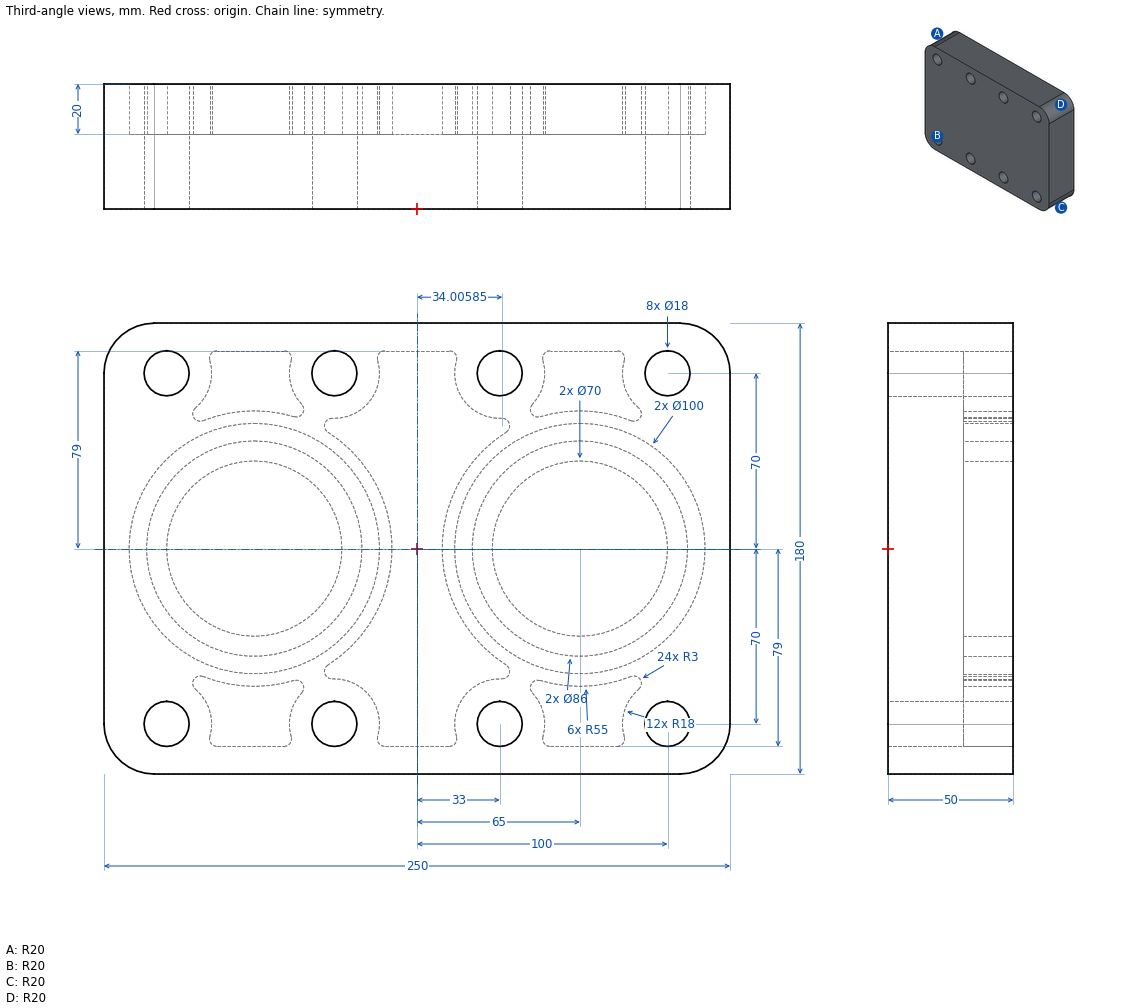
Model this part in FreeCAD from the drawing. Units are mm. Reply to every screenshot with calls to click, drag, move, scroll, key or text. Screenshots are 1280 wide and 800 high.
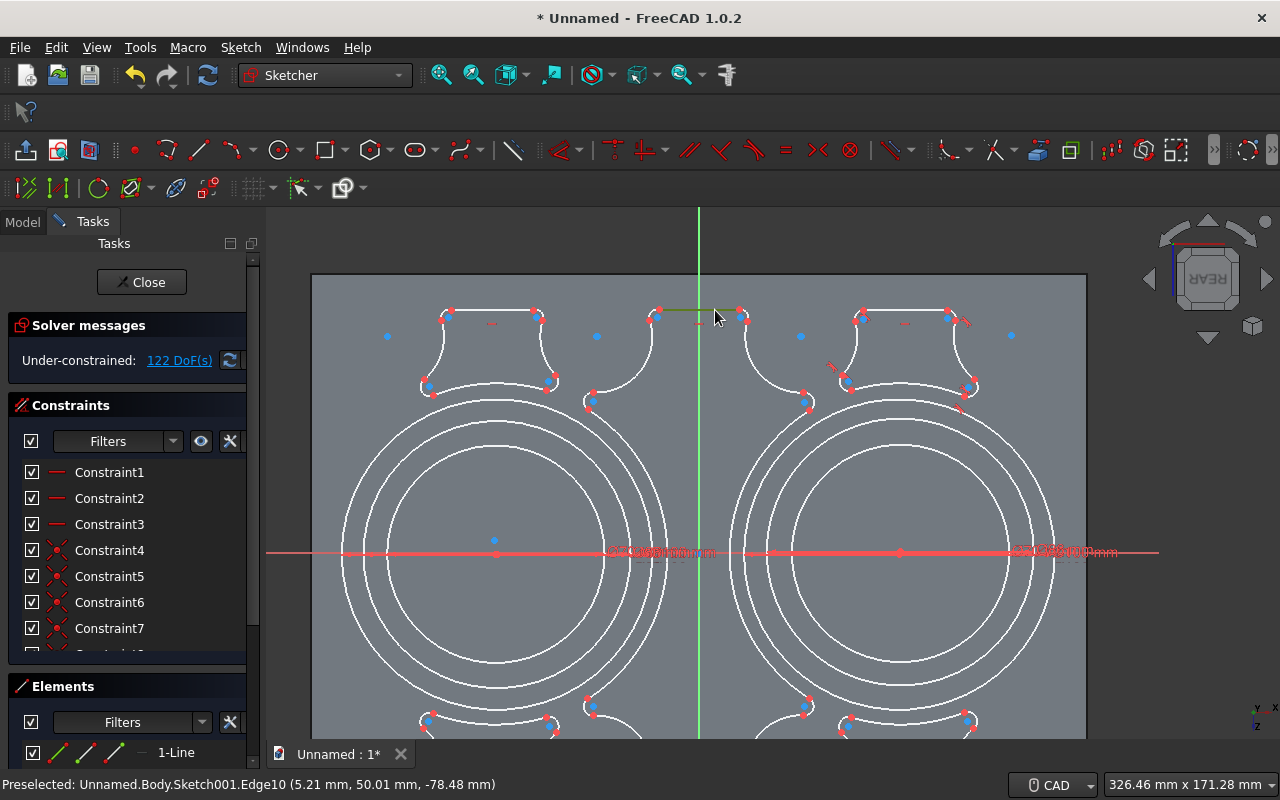
scroll(747, 313, up, 3)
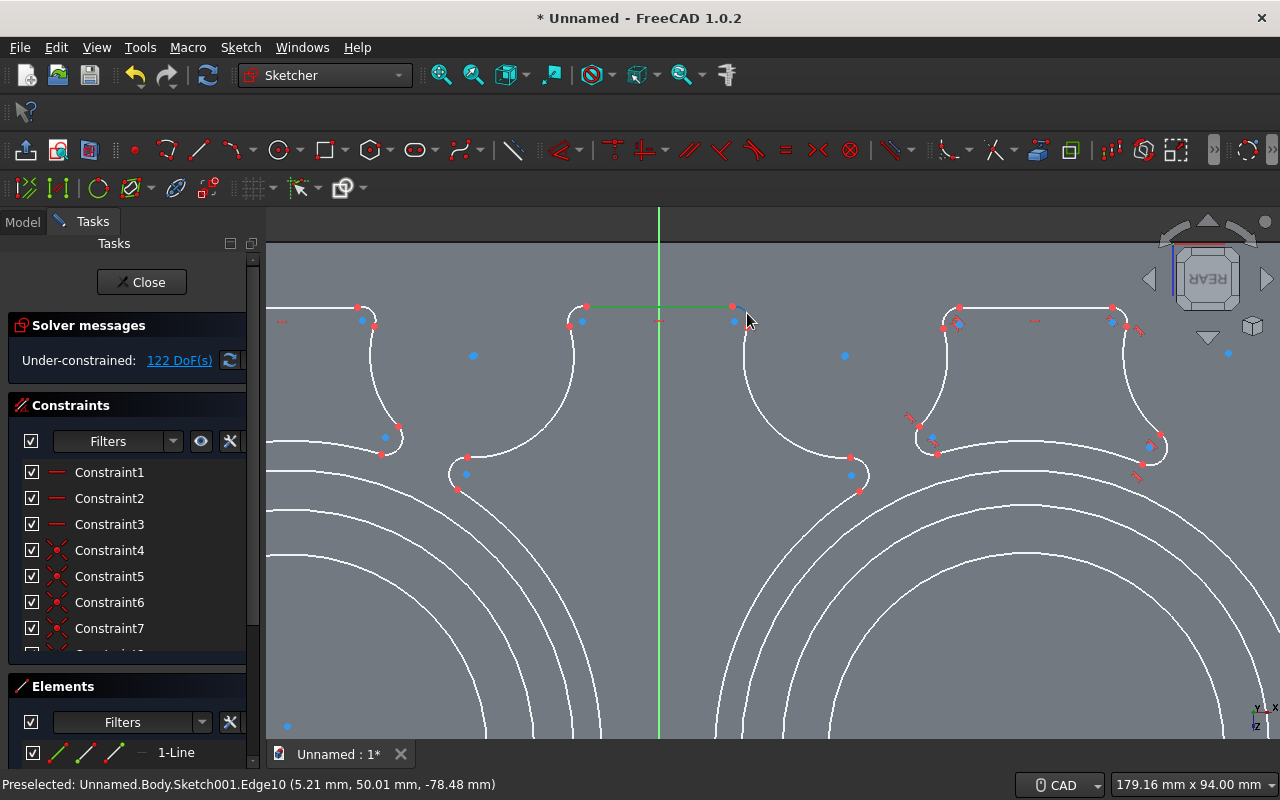
click(747, 313)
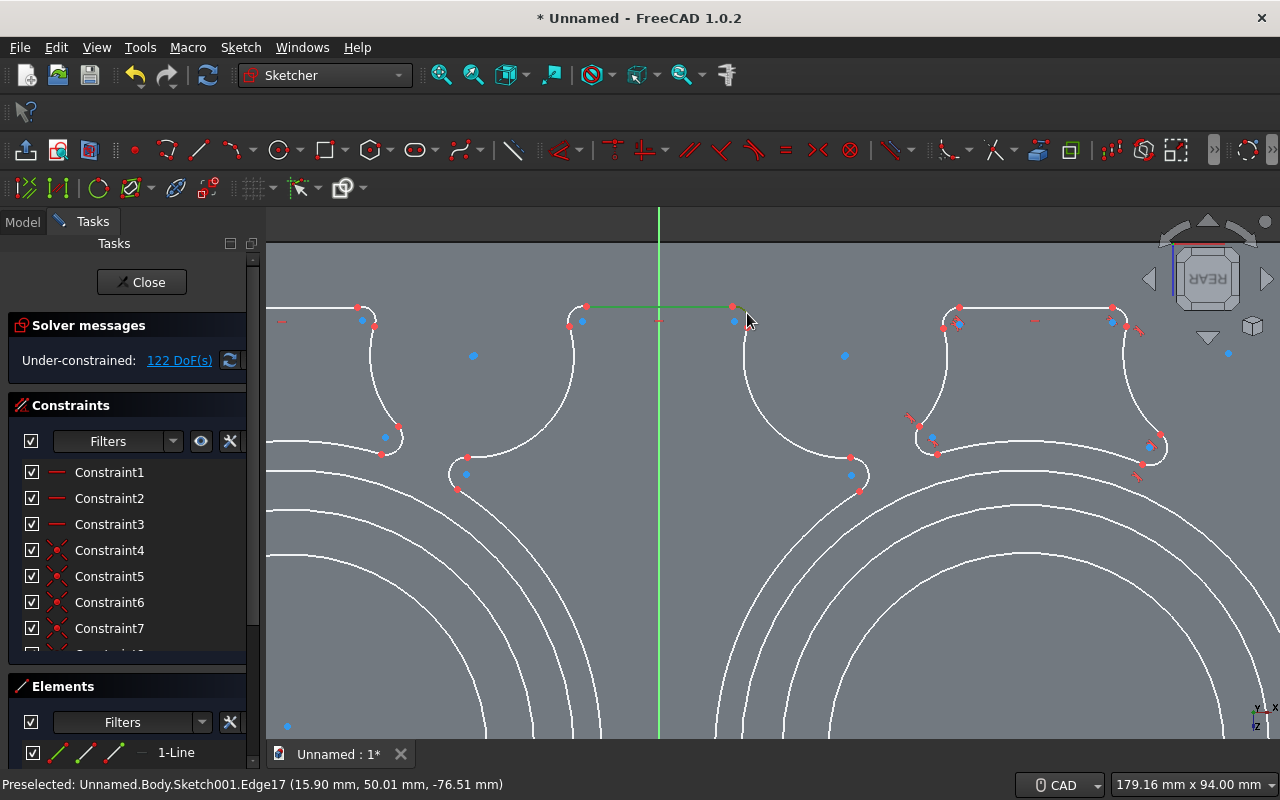
click(754, 150)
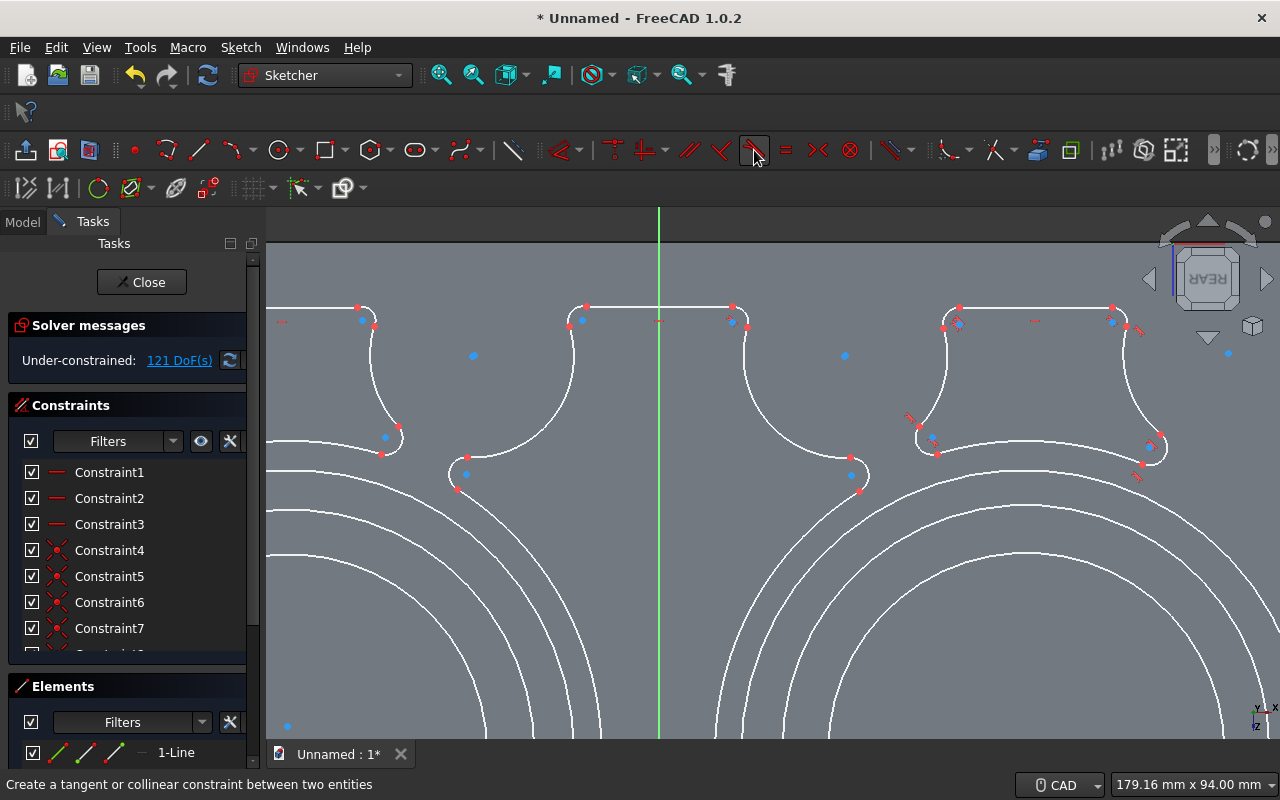
click(689, 307)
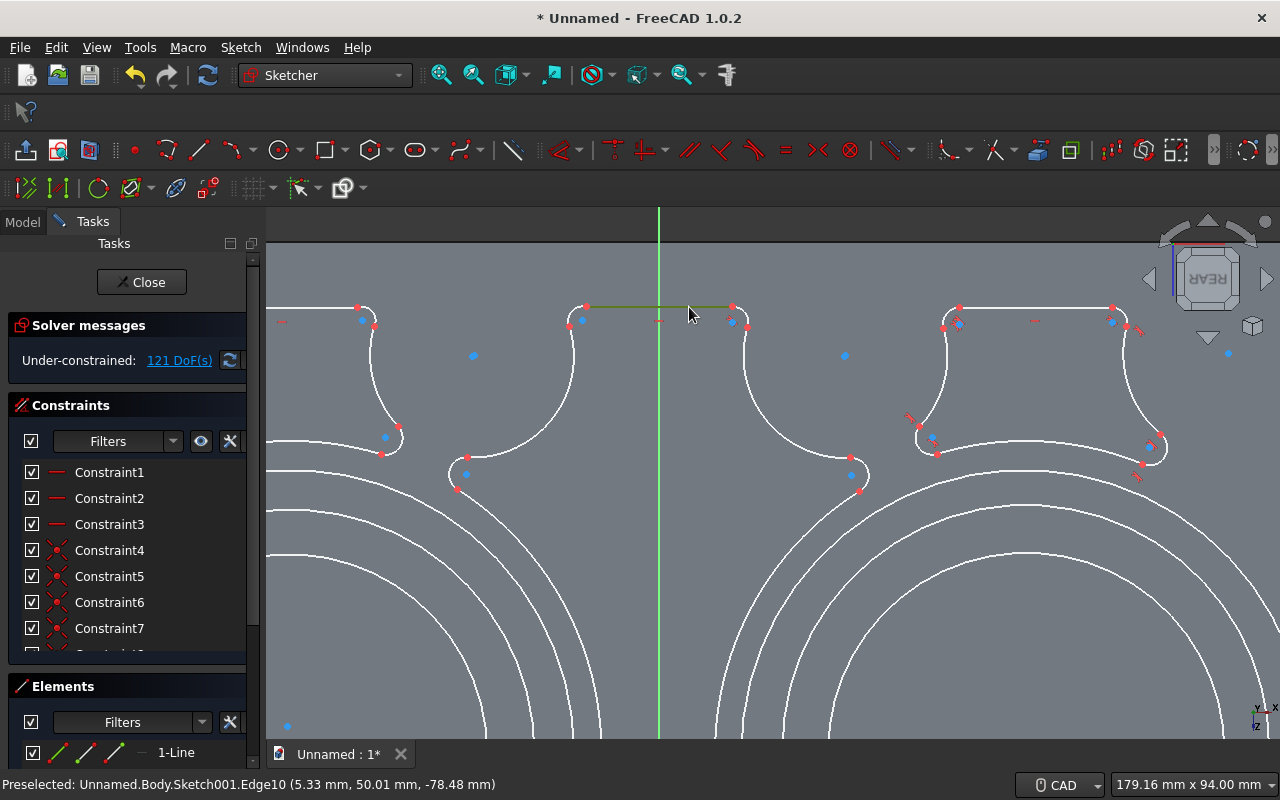
scroll(577, 308, up, 2)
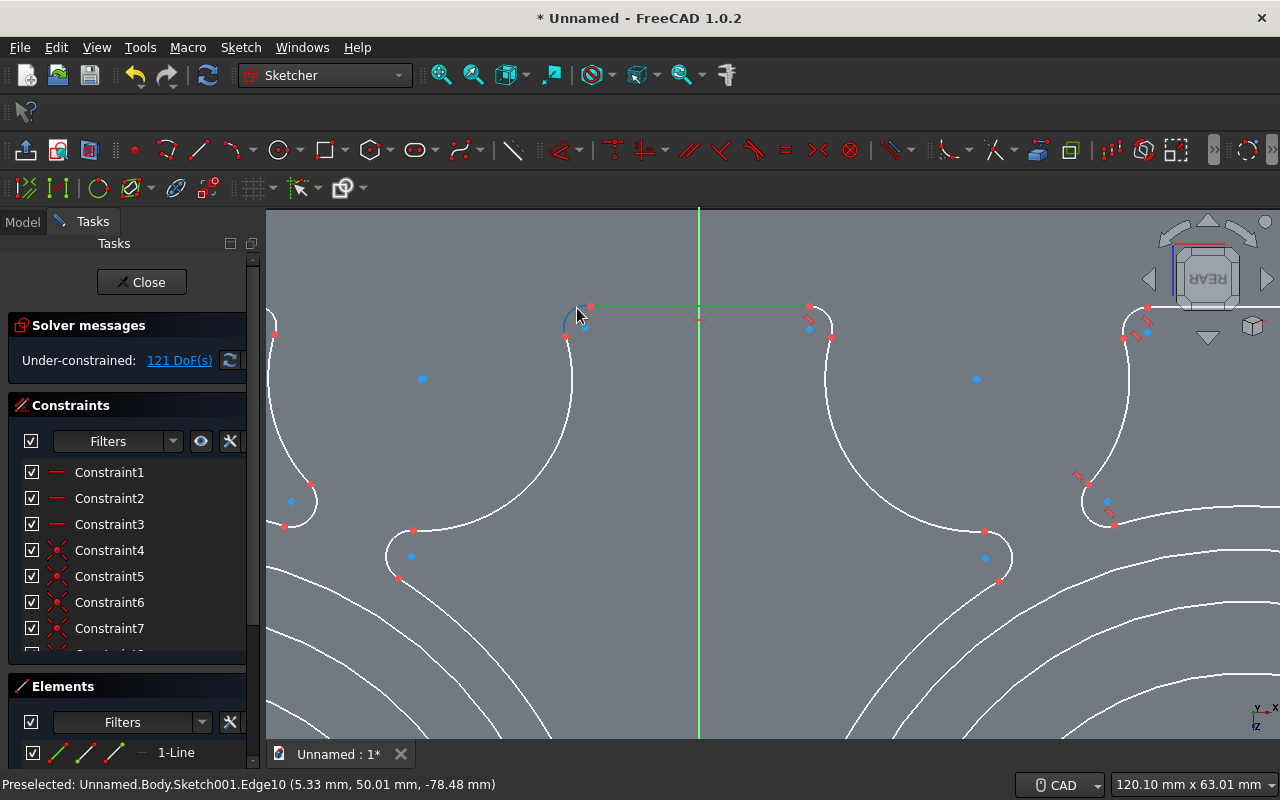
click(577, 307)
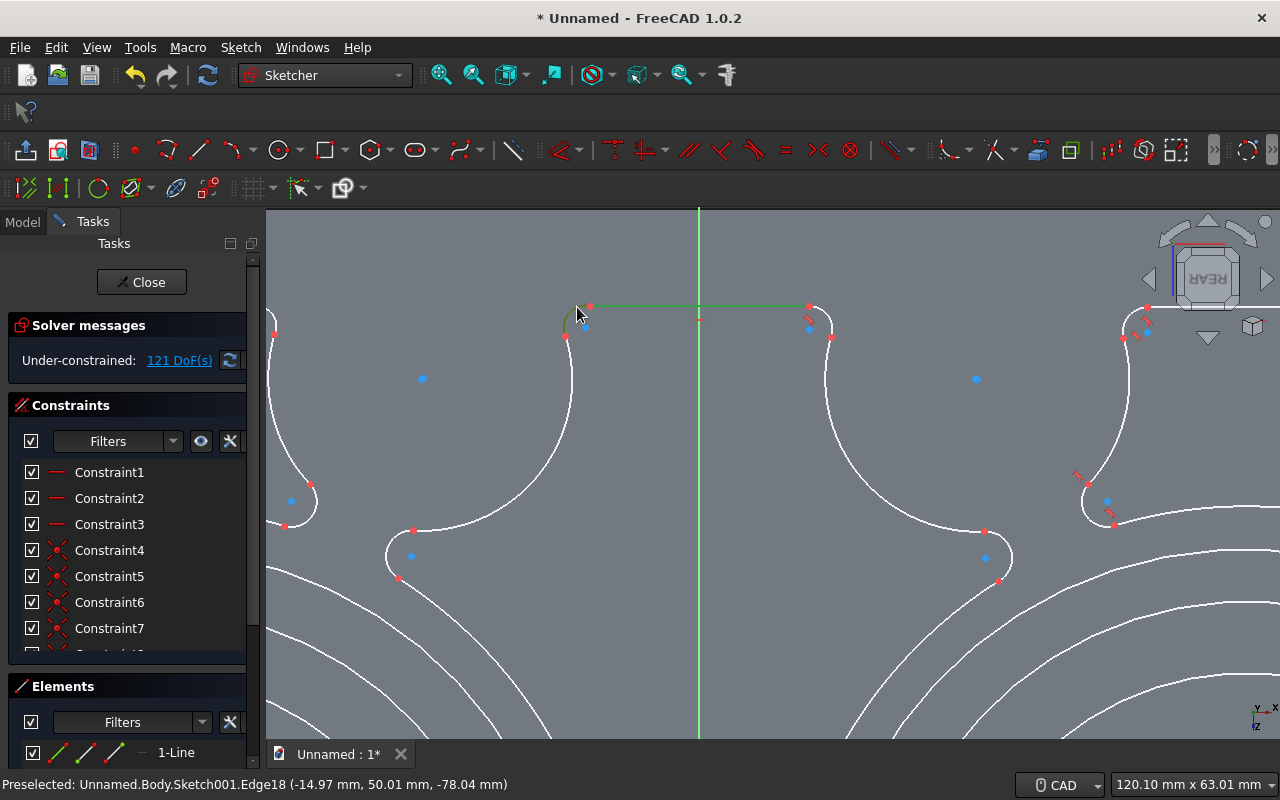
click(754, 150)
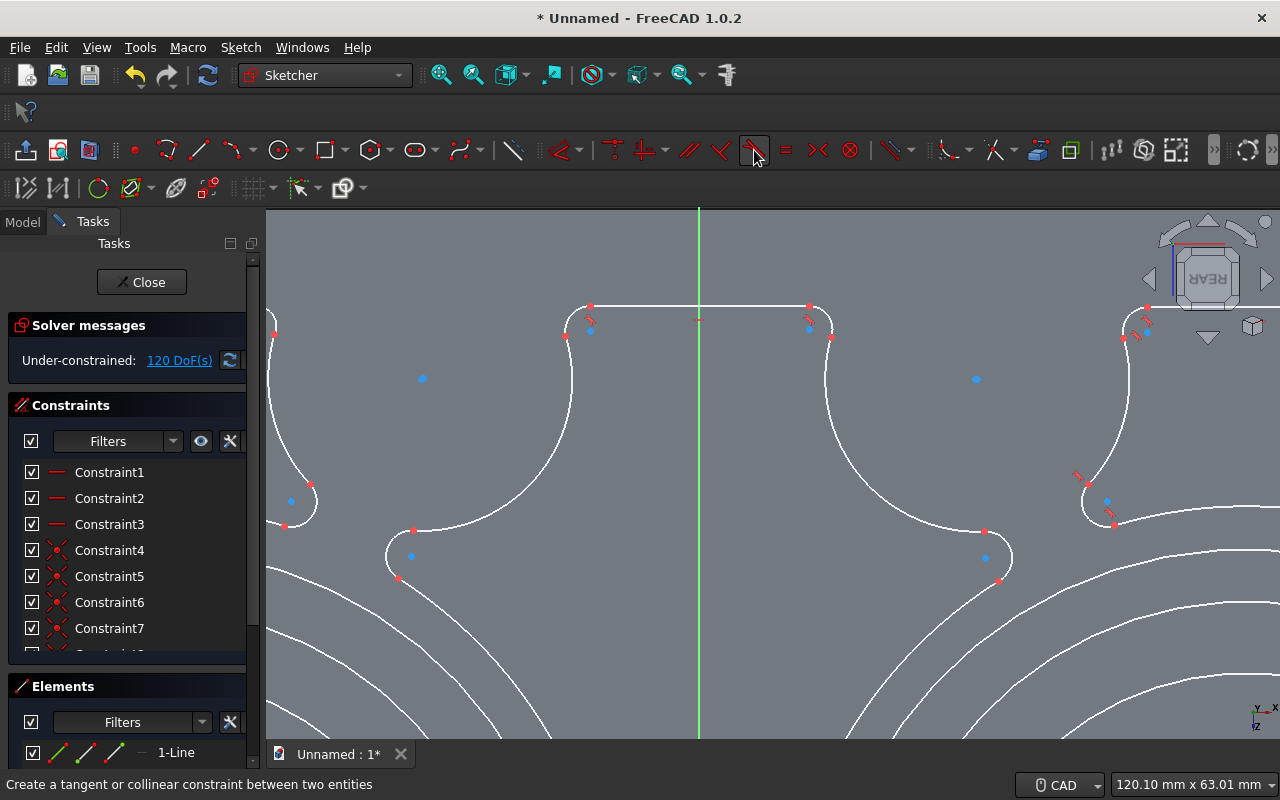
scroll(706, 311, down, 7)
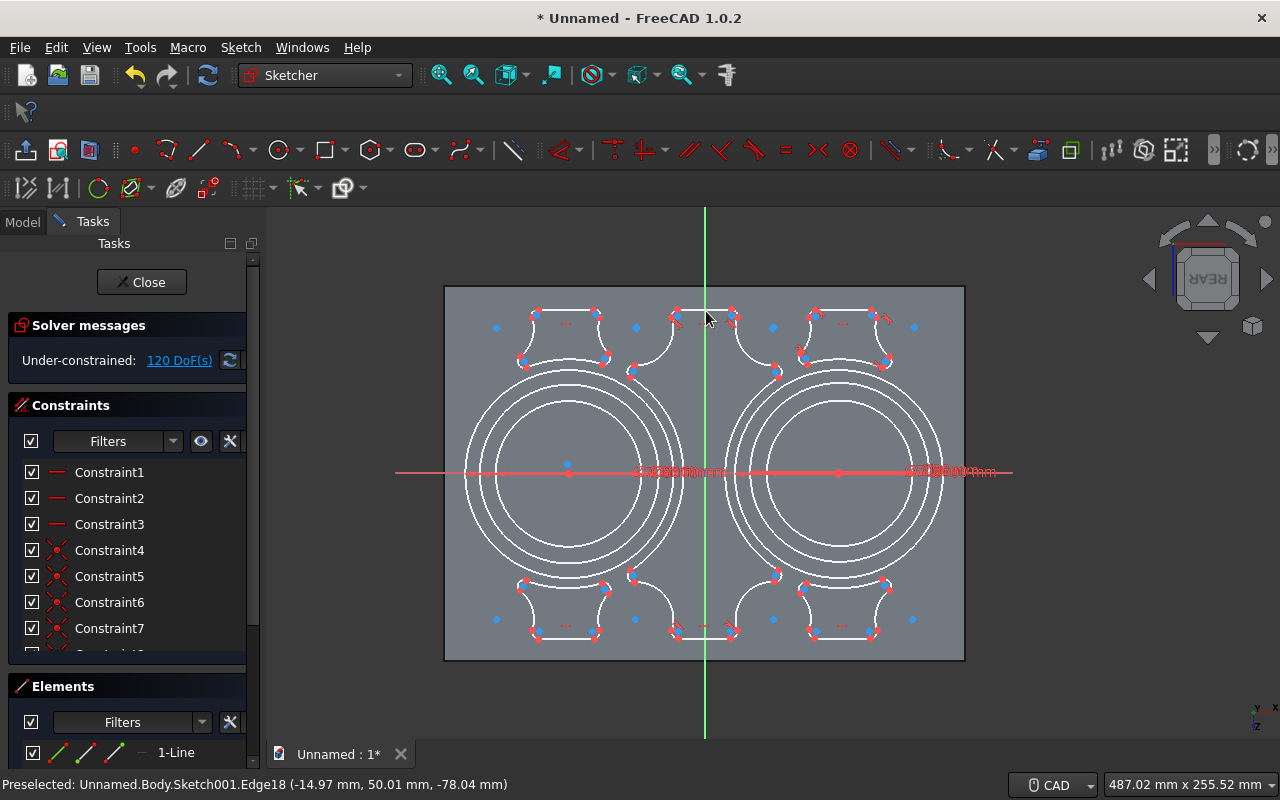
scroll(734, 638, up, 7)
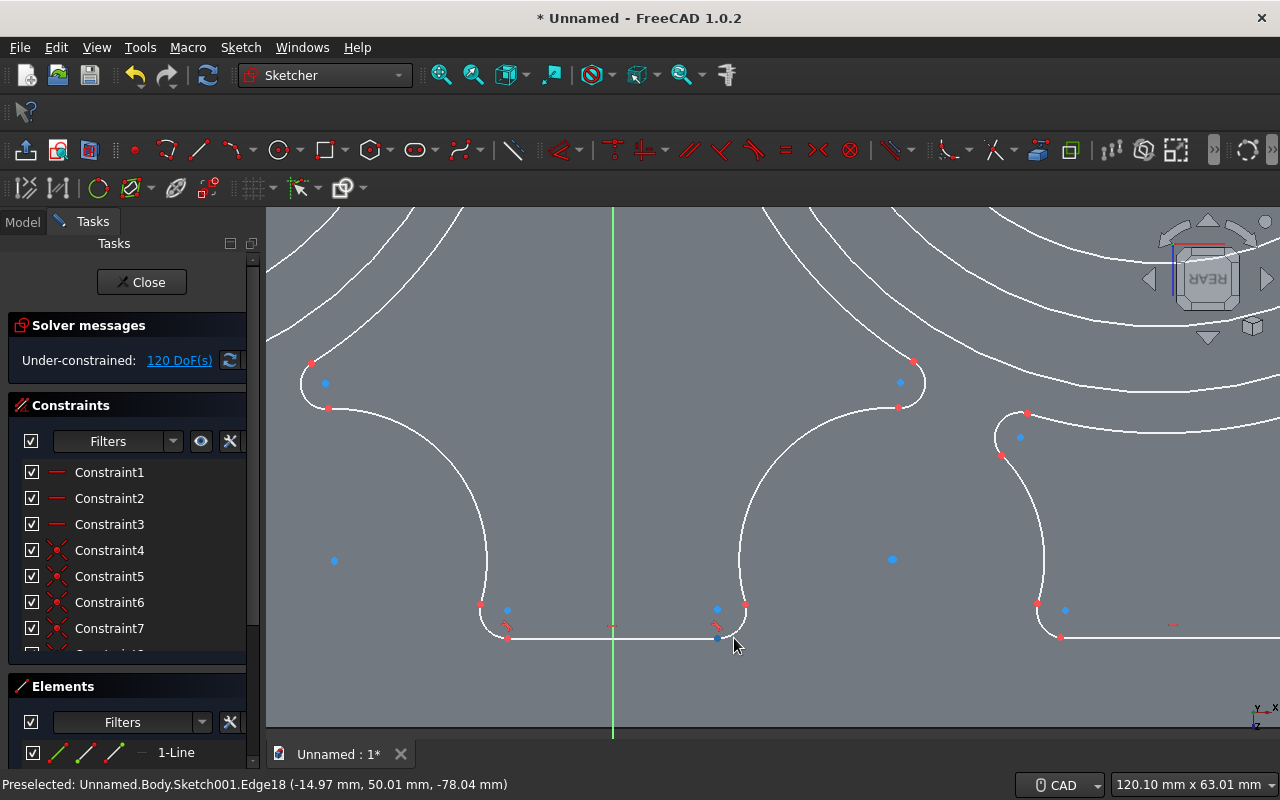
click(732, 635)